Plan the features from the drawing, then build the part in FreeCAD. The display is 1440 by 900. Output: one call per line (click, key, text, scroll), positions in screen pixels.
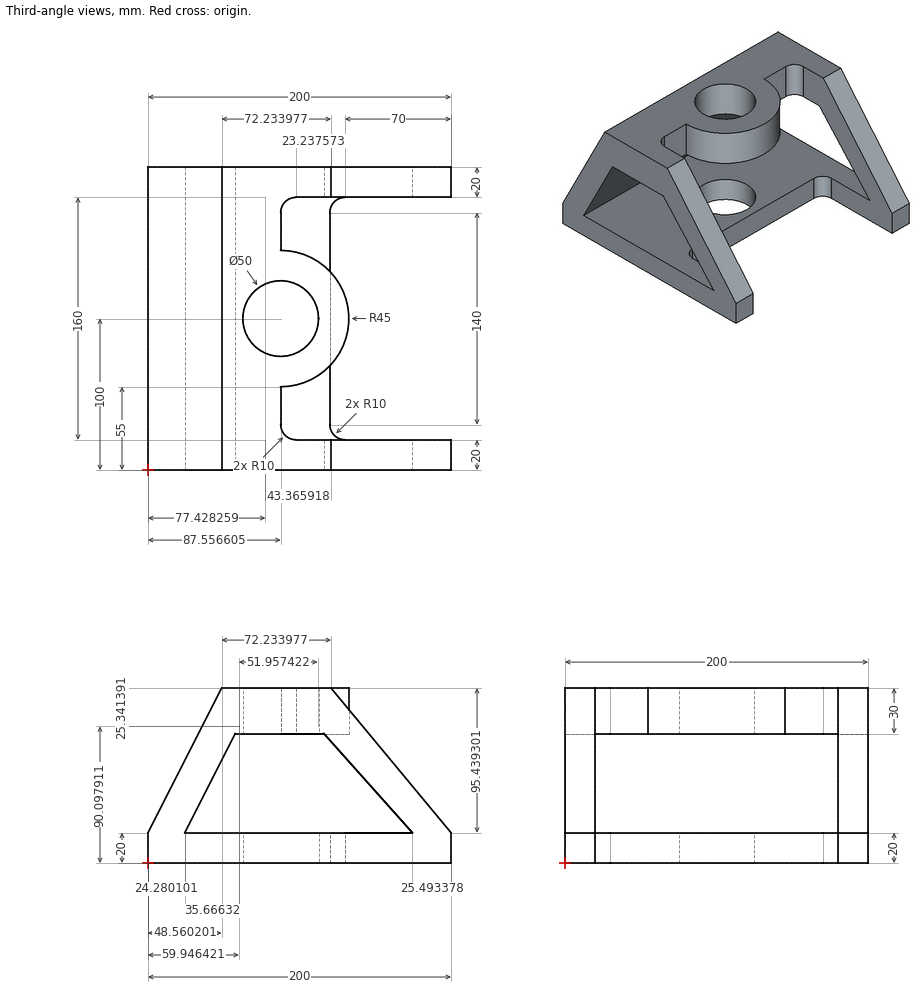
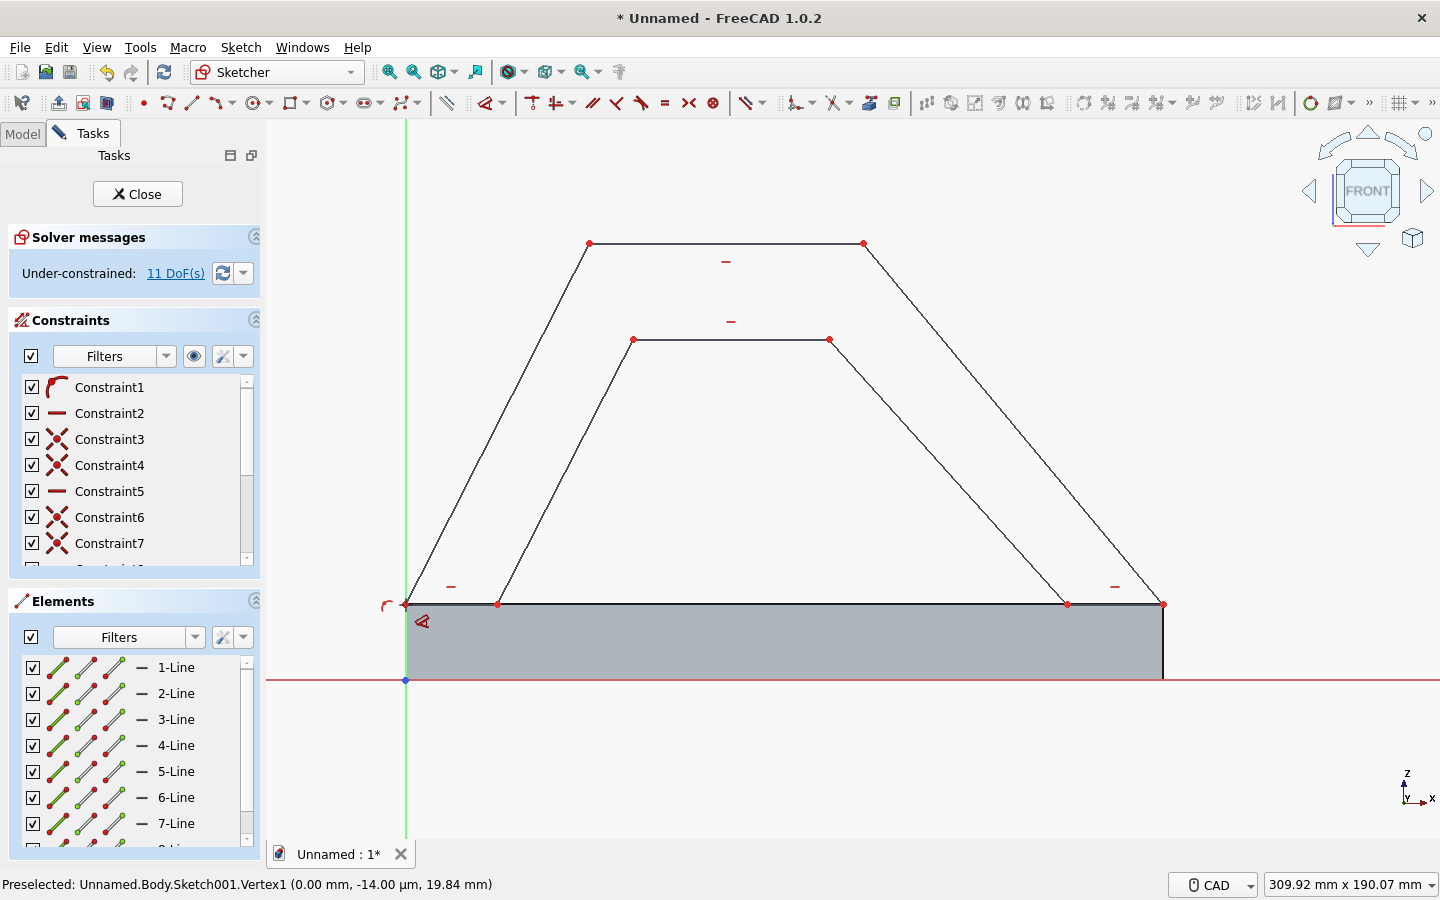
click(406, 605)
click(372, 643)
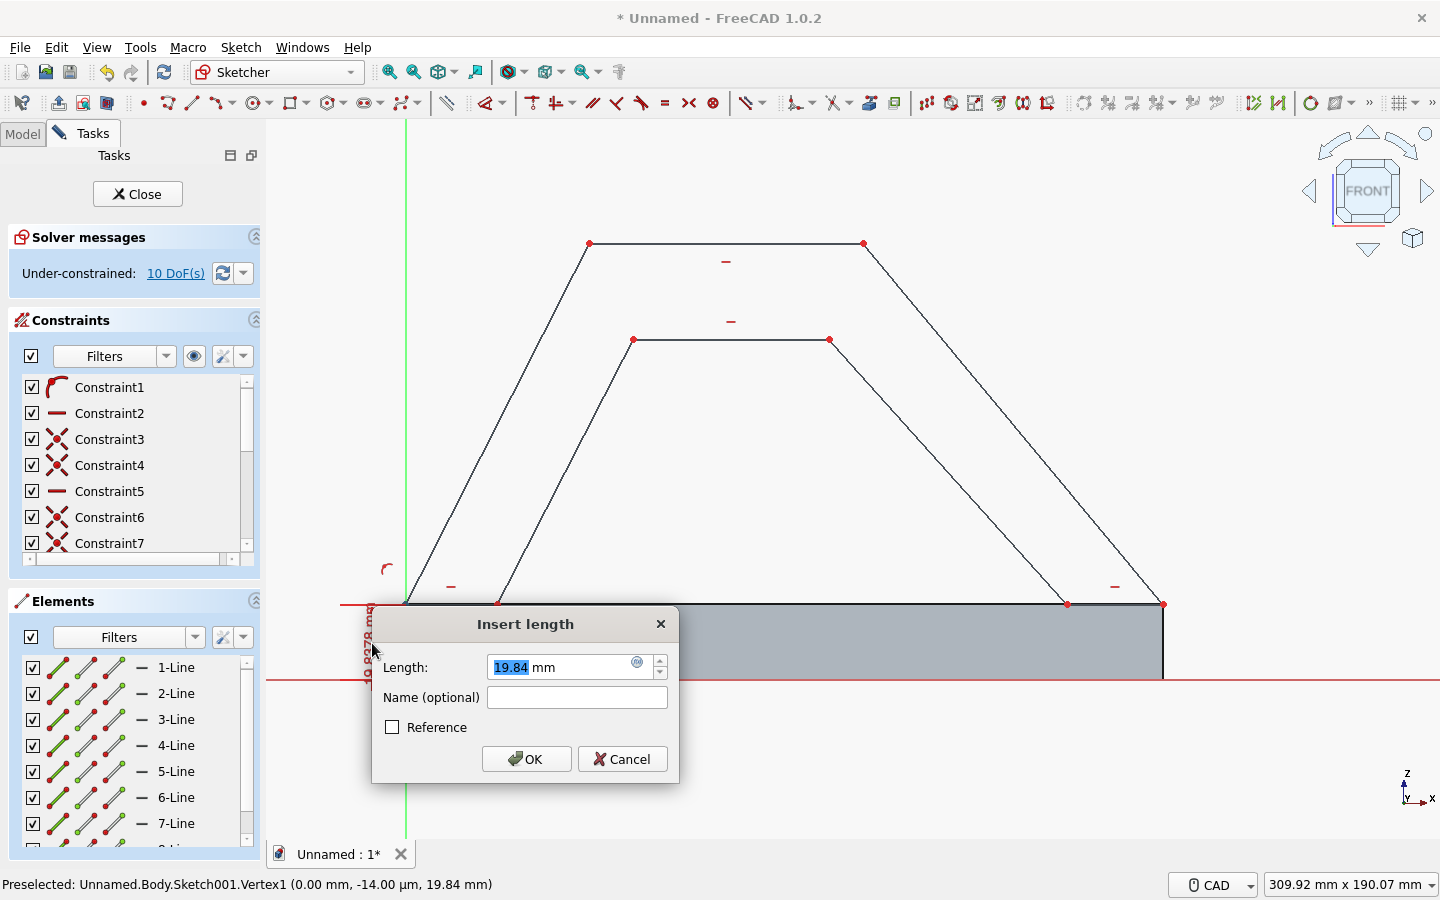
text(20)
key(Return)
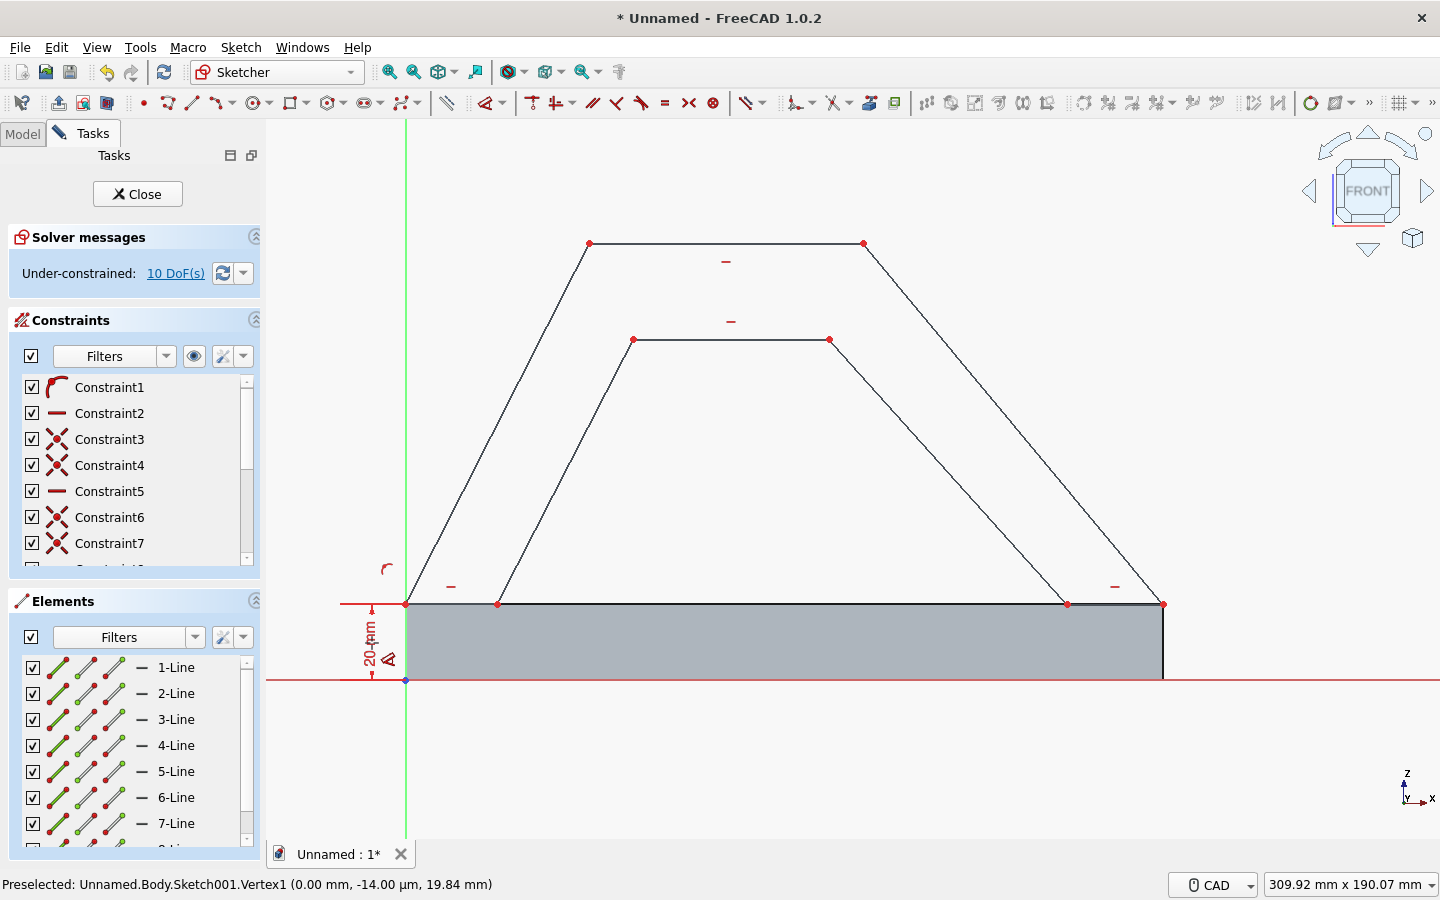
click(1067, 605)
click(372, 616)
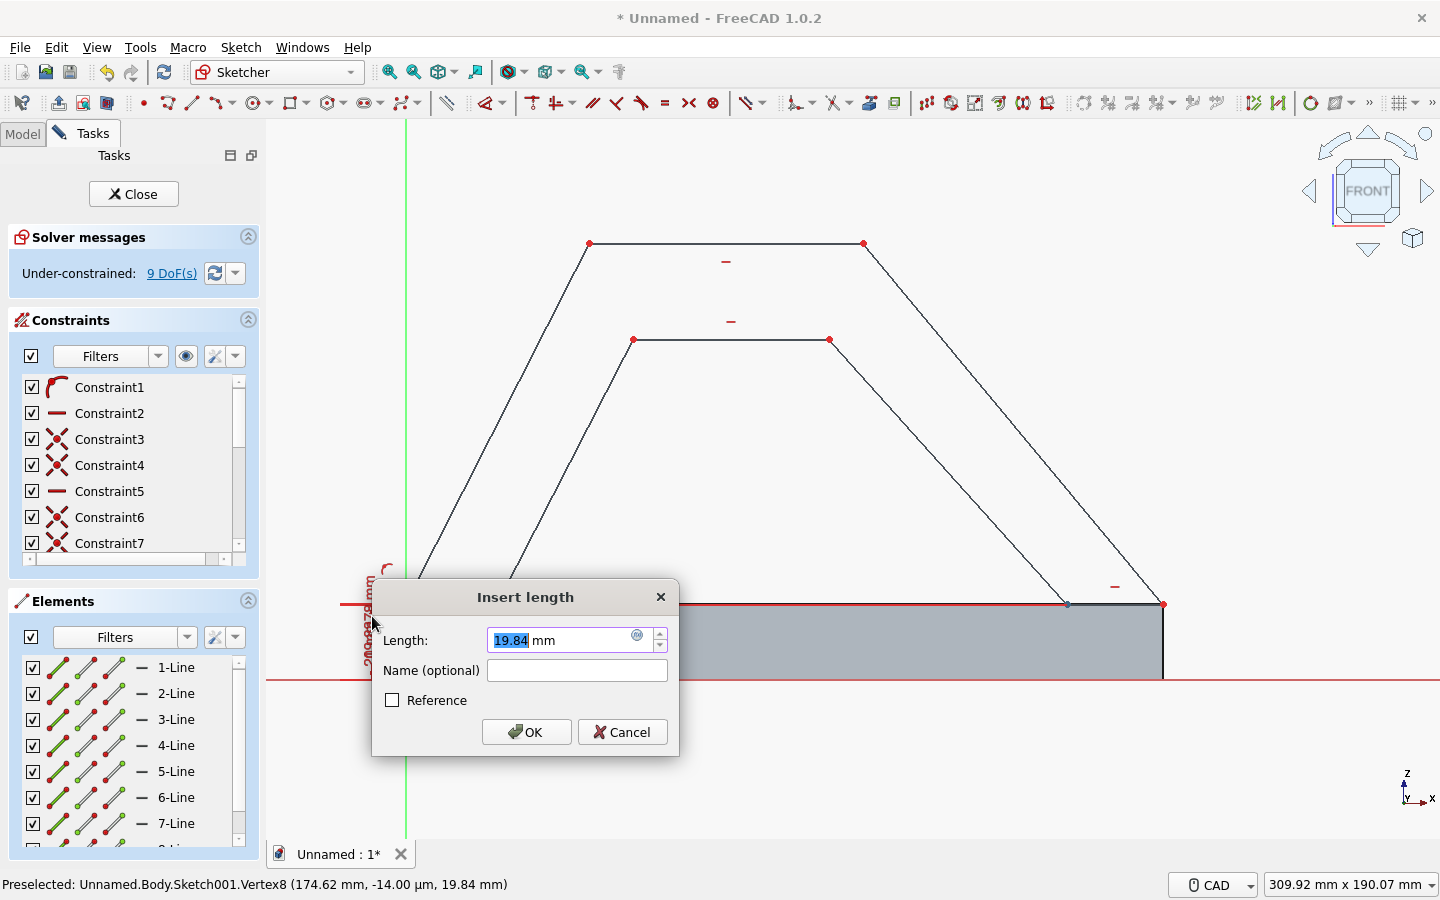
text(20)
key(Return)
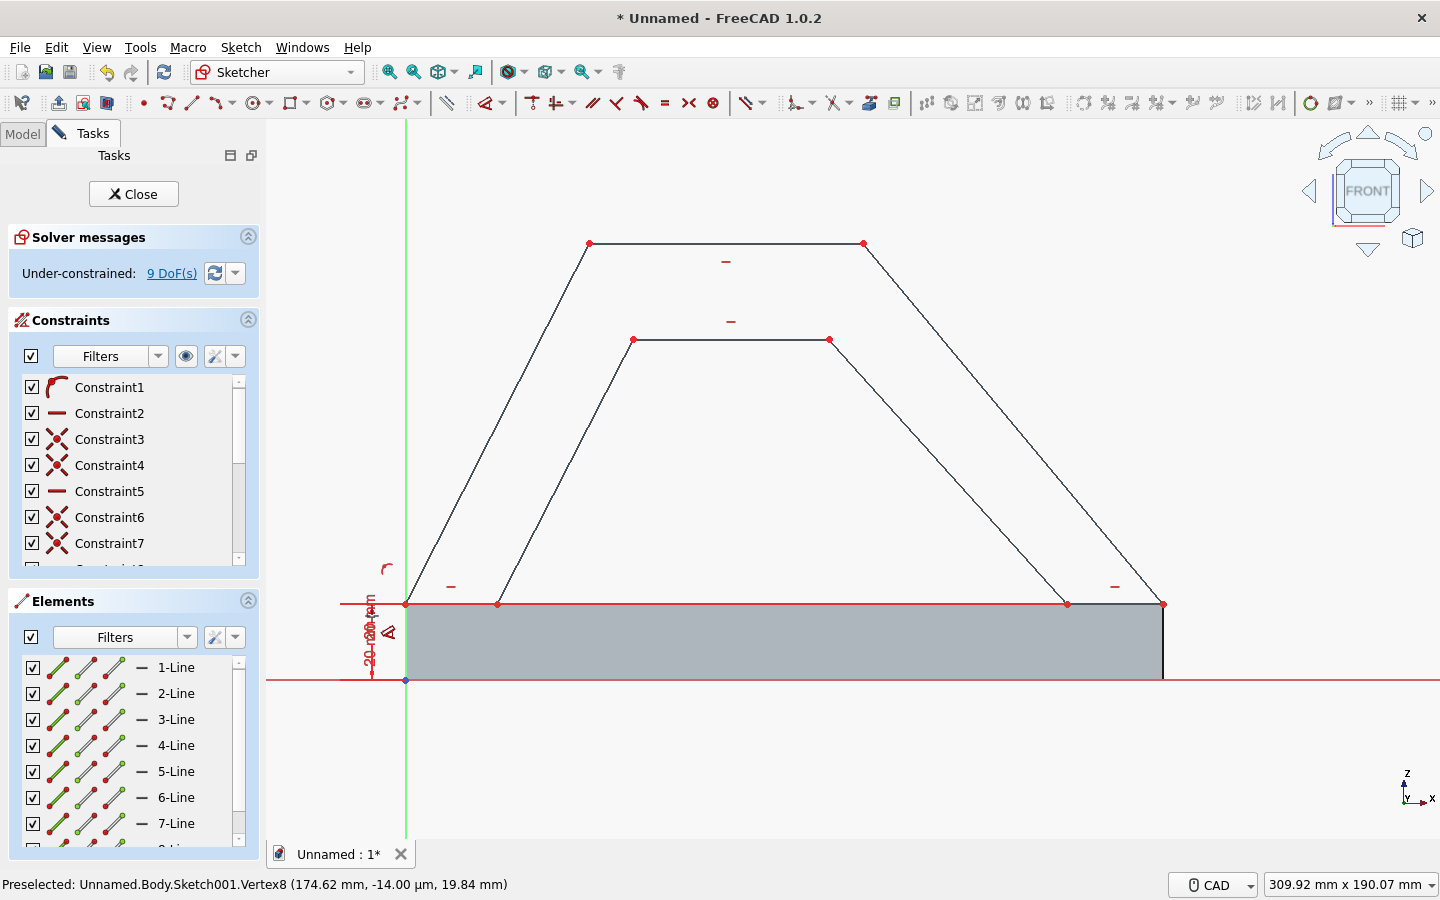
click(1163, 604)
click(784, 714)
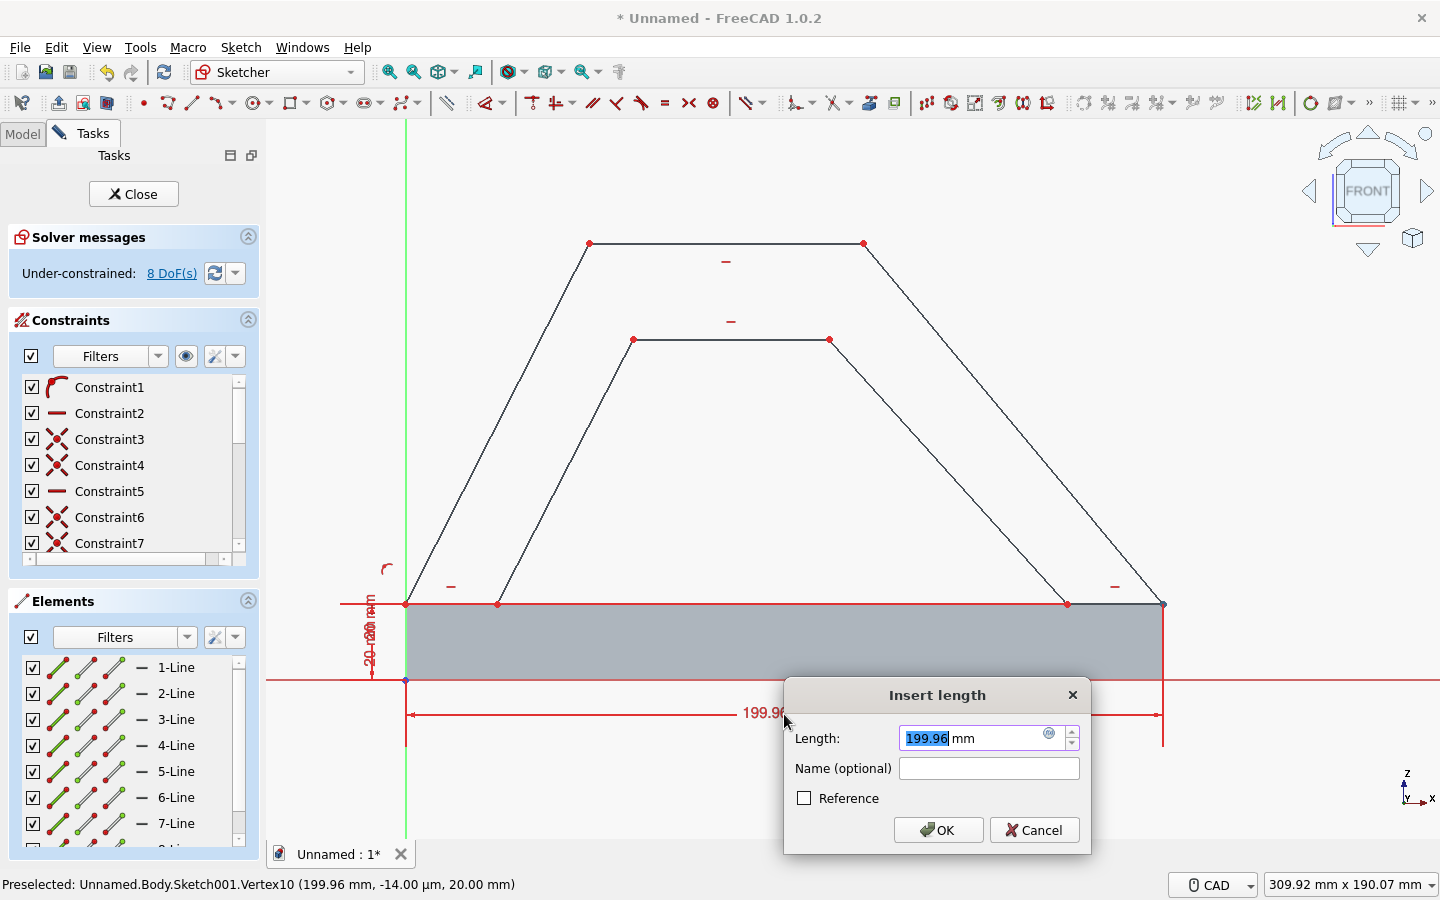
text(200)
key(Return)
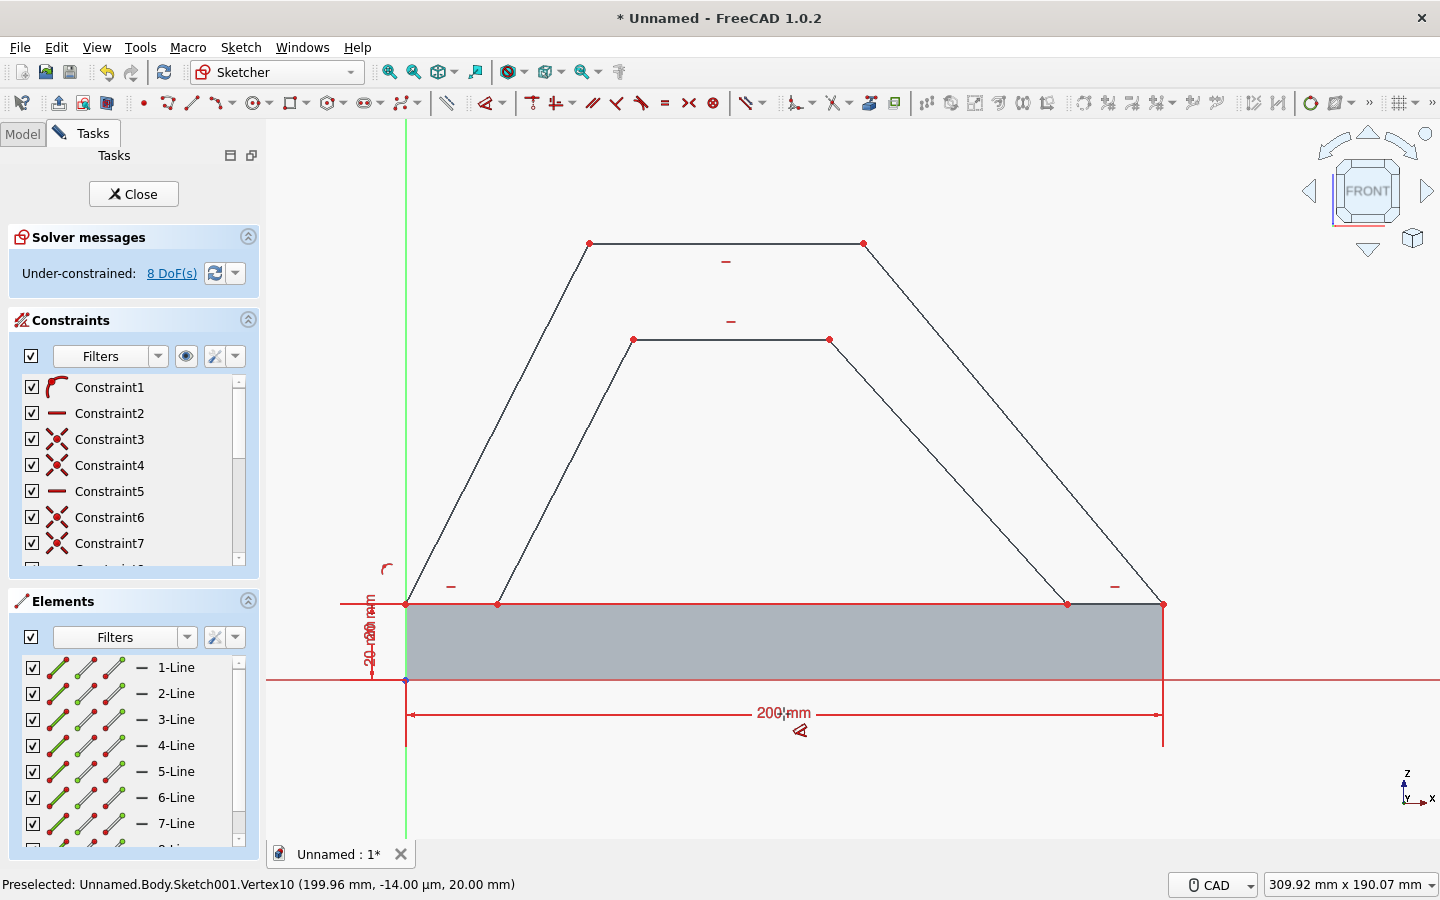
click(433, 604)
click(451, 638)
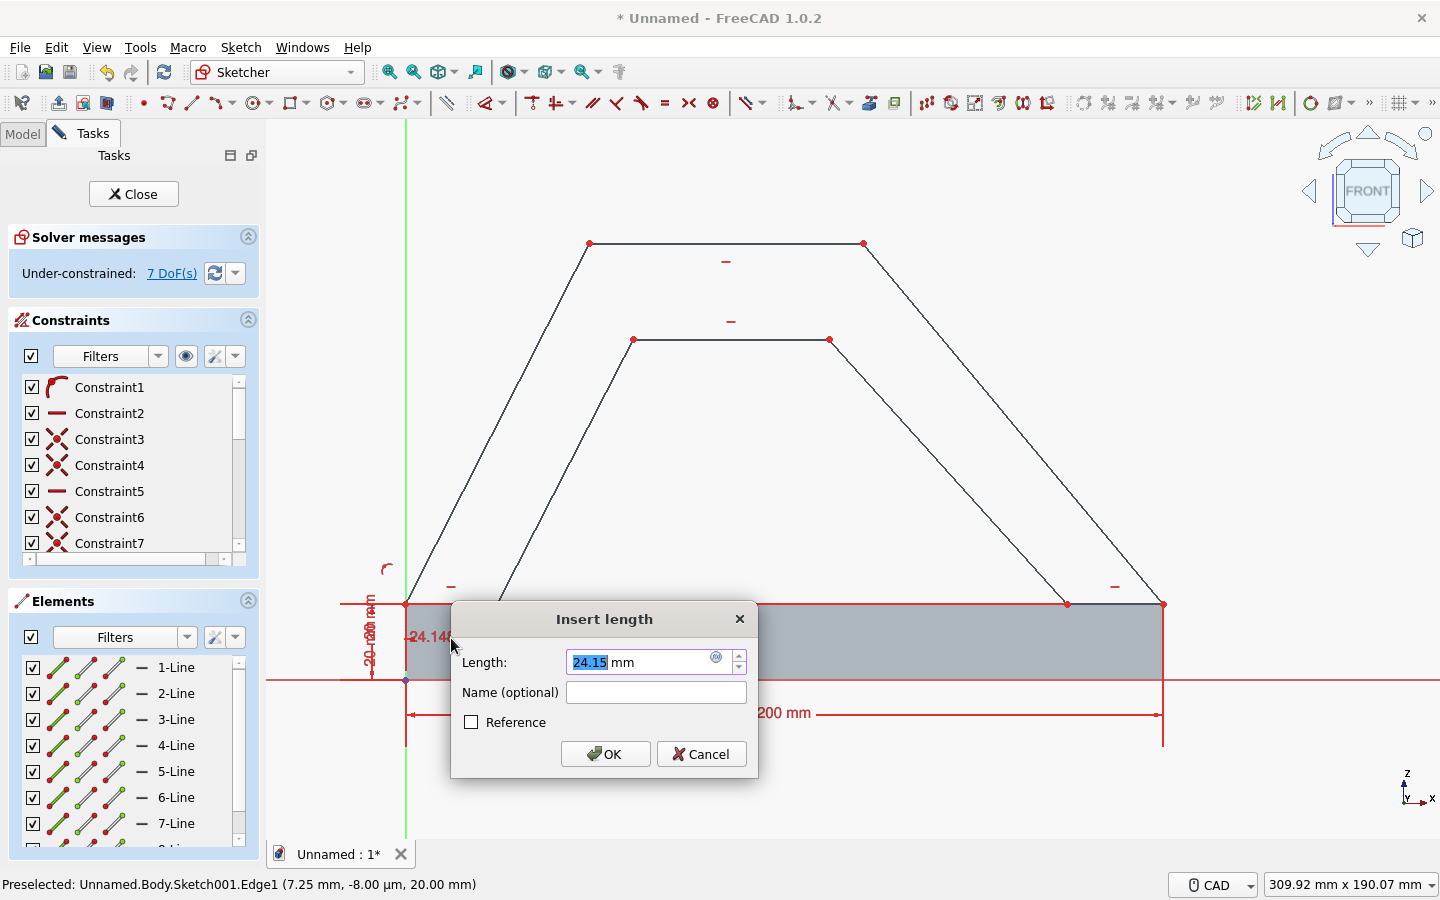
text(24.280101)
key(Return)